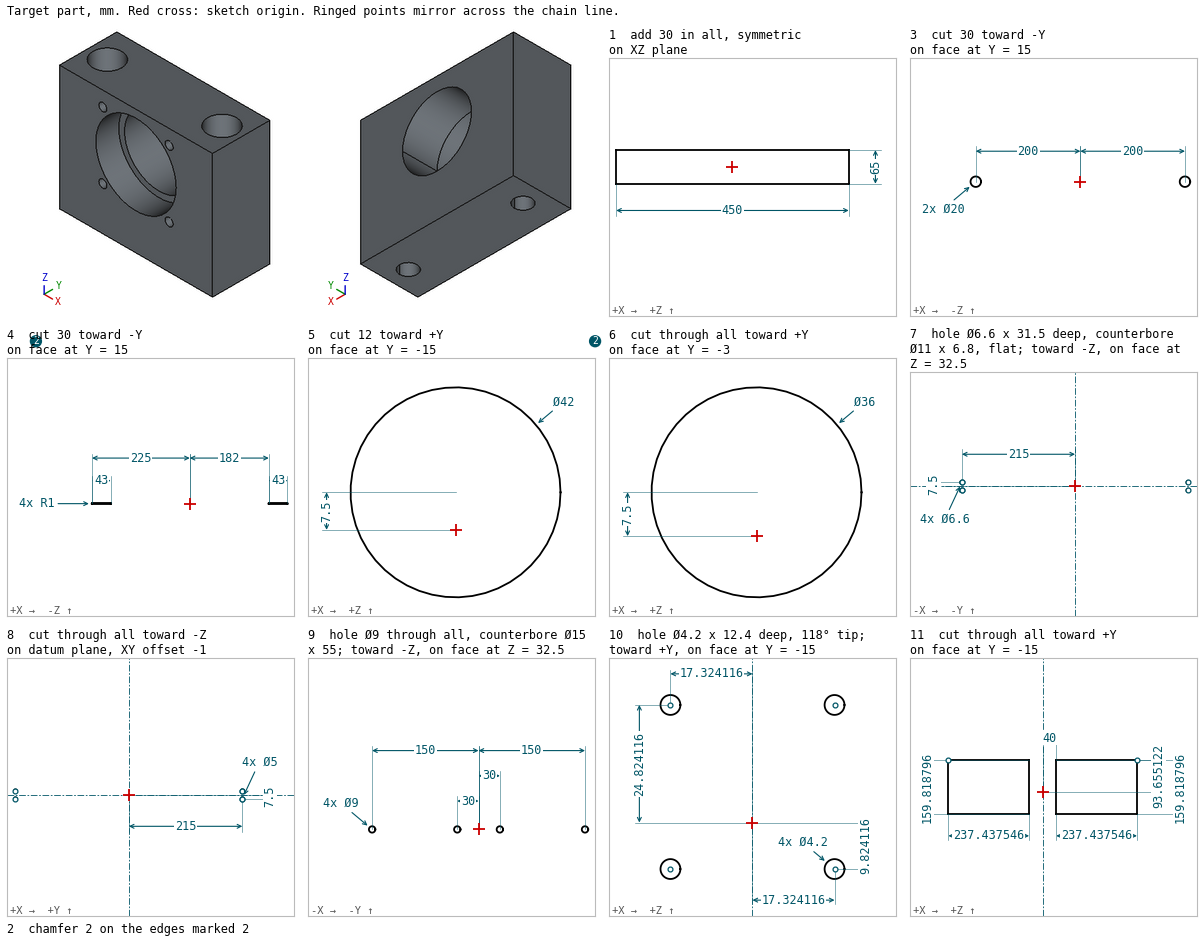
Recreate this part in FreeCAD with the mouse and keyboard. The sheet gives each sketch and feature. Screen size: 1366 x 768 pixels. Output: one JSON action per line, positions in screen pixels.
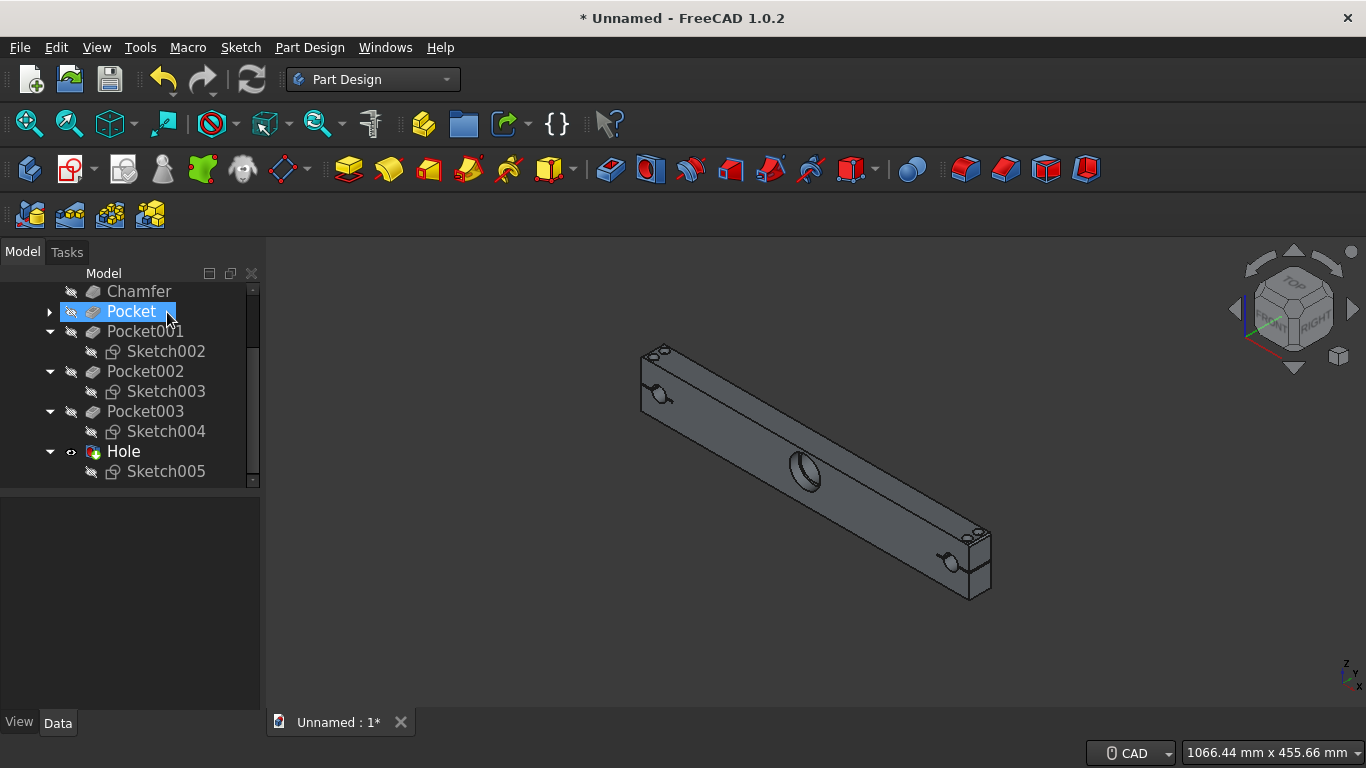
{"action": "key", "text": "1"}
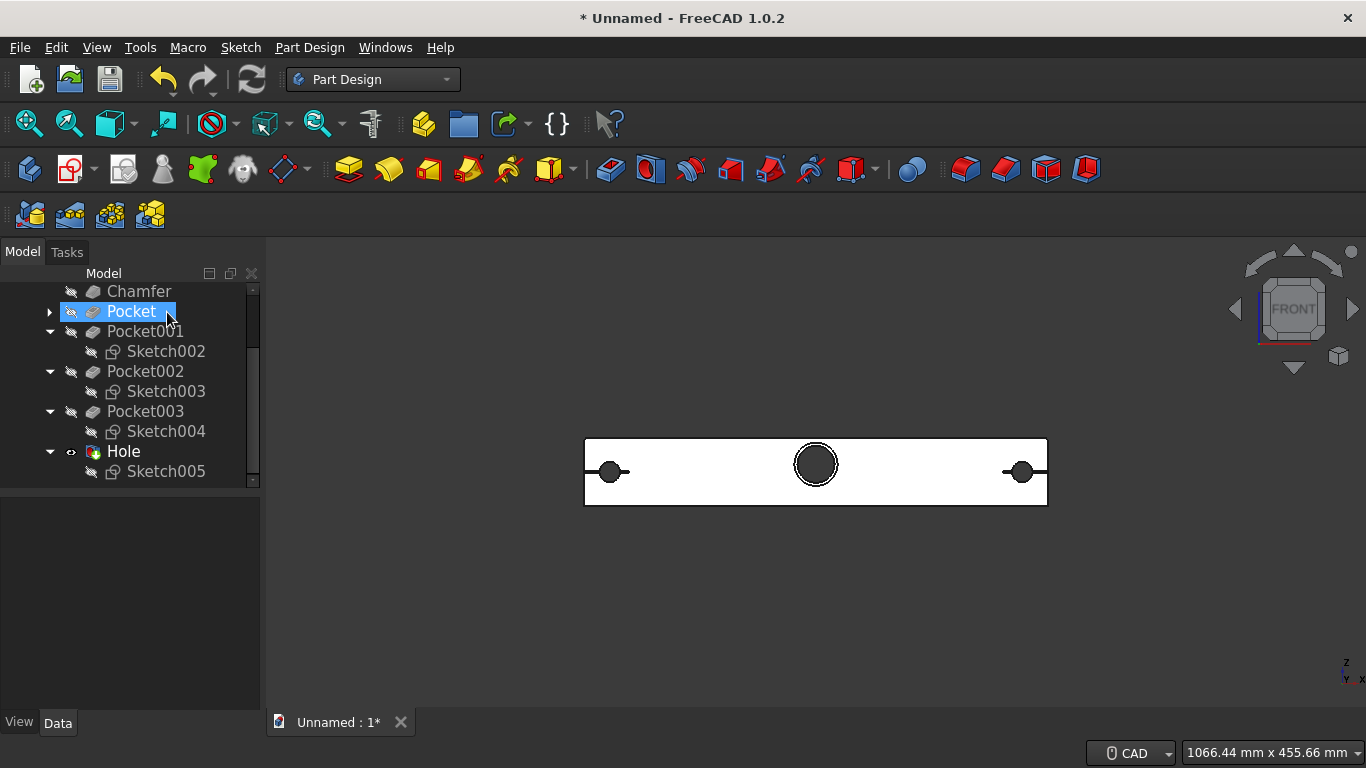
{"action": "key", "text": "v f"}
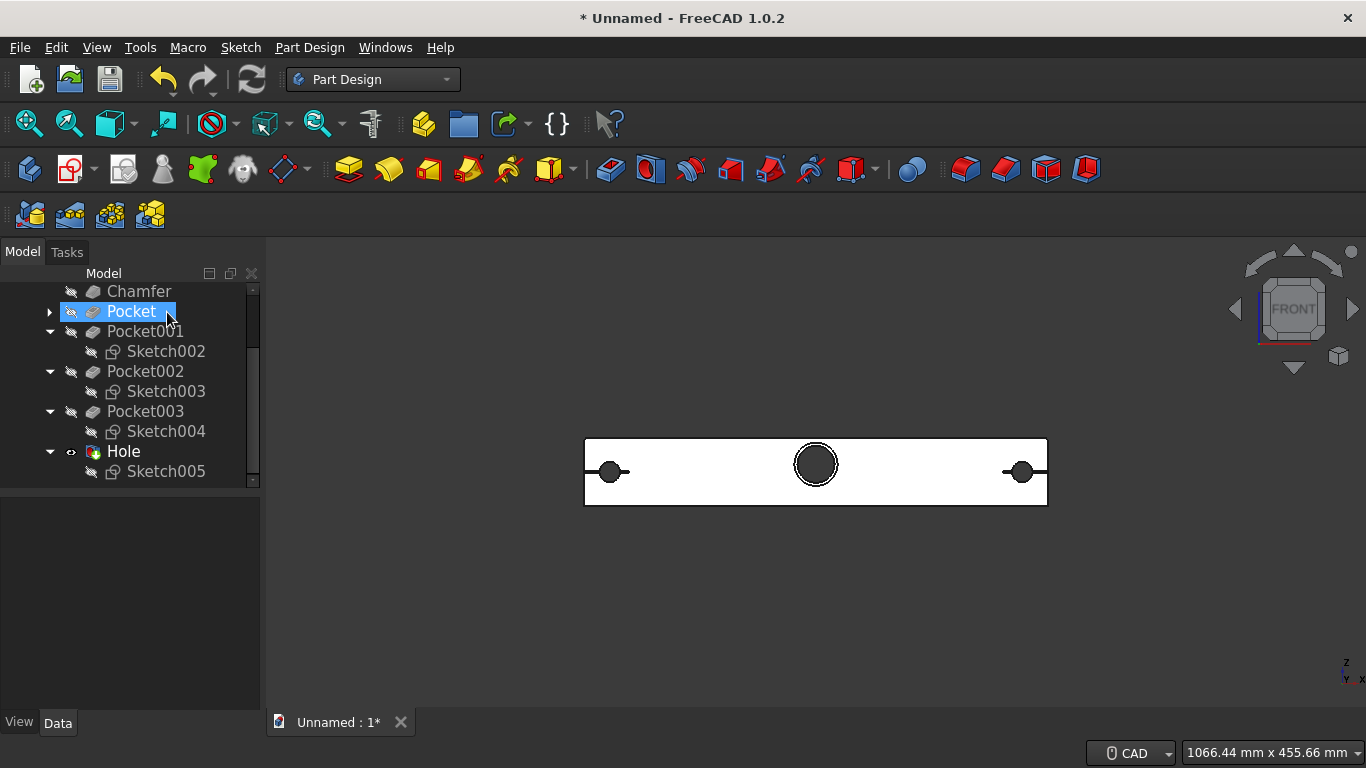
{"action": "scroll", "coordinate": [140, 387], "scroll_direction": "down", "scroll_amount": 3}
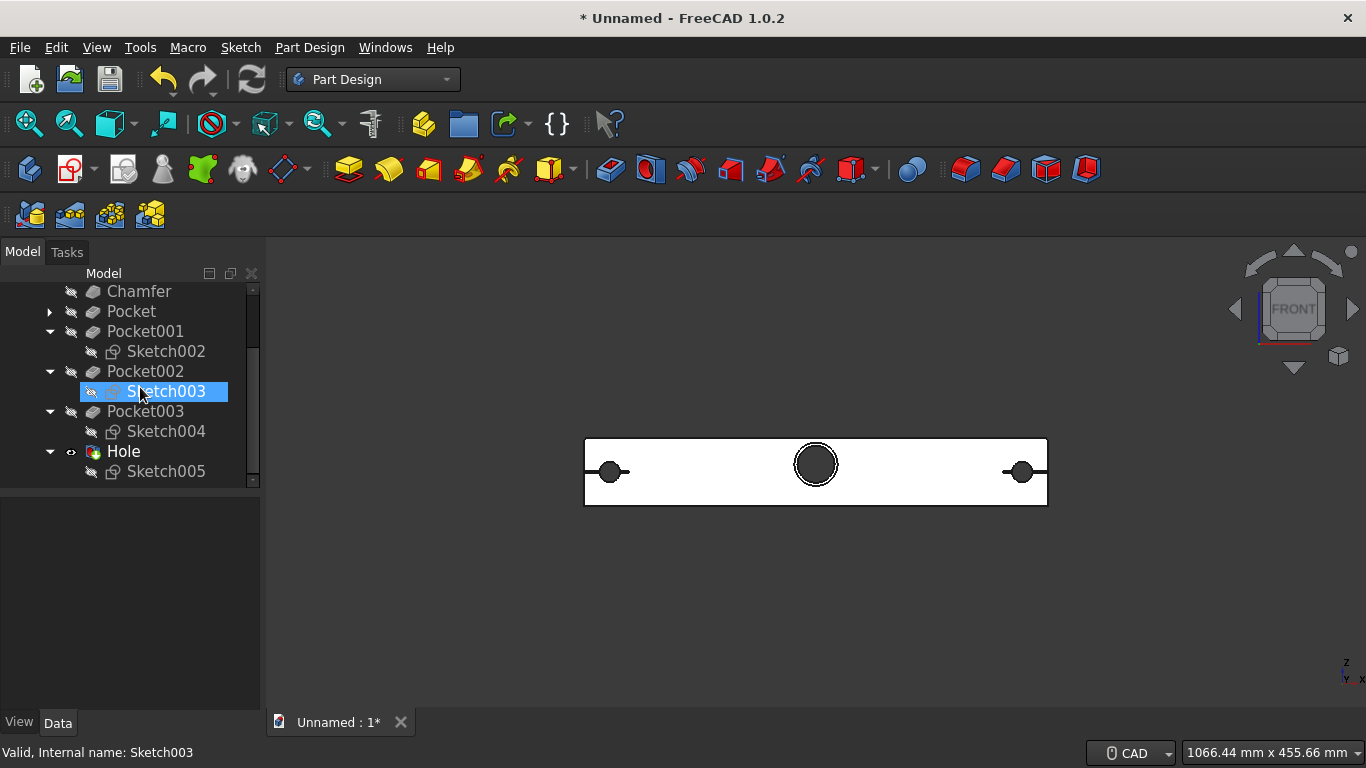
{"action": "scroll", "coordinate": [140, 387], "scroll_direction": "up", "scroll_amount": 15}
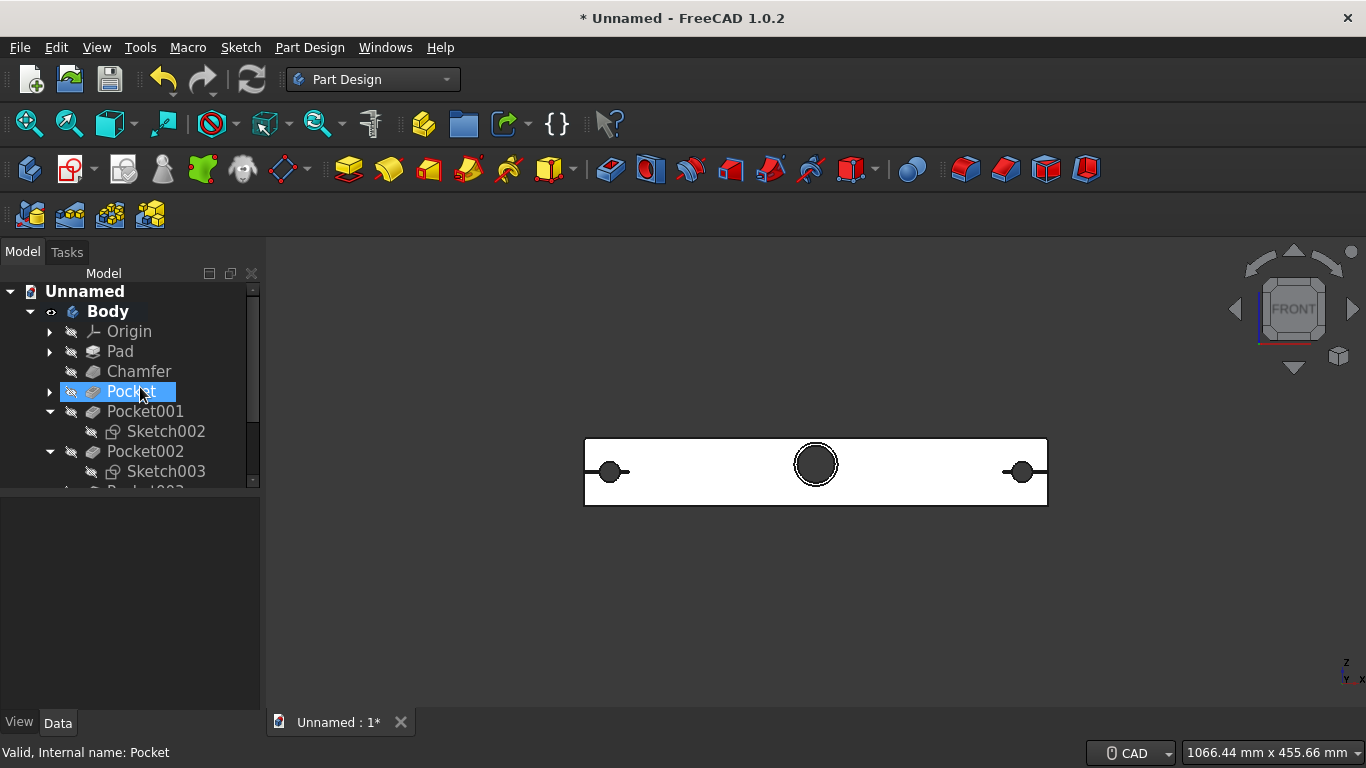
{"action": "left_click", "coordinate": [50, 332]}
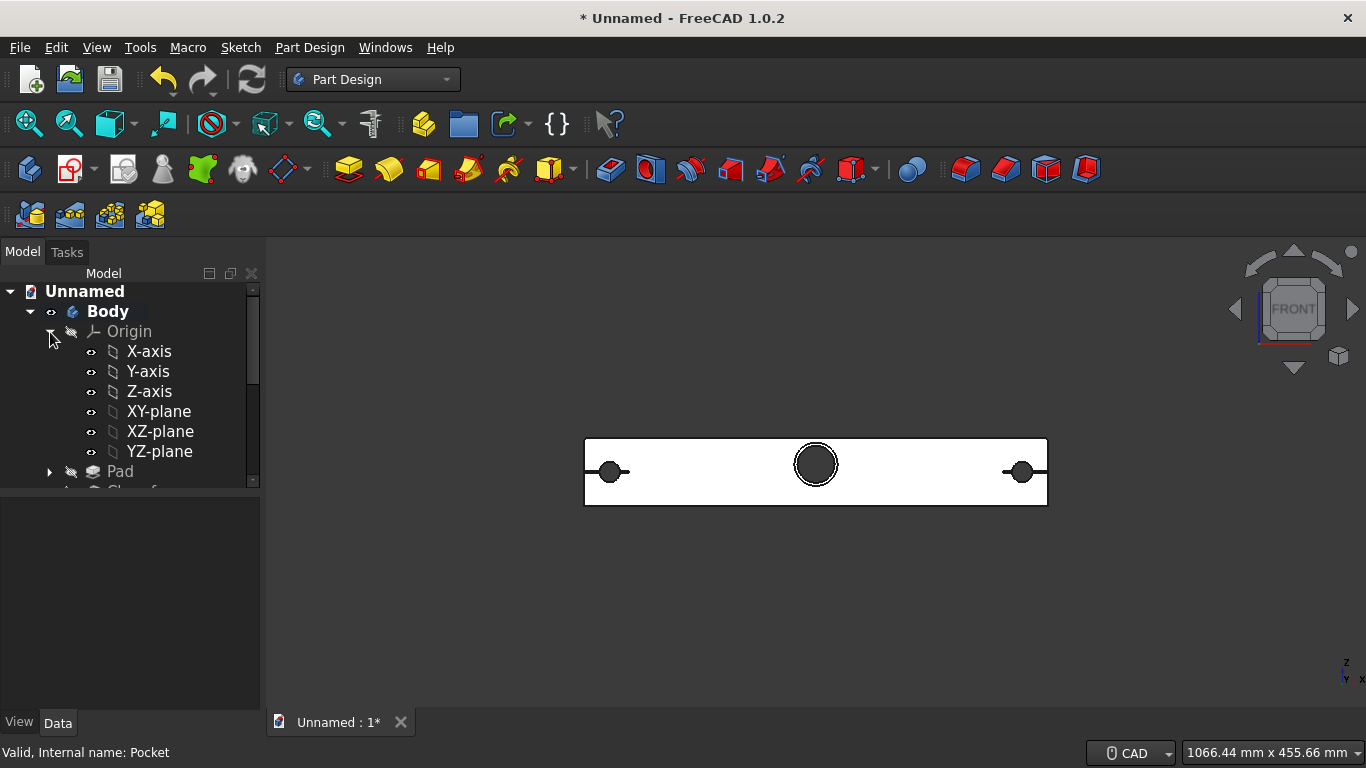
{"action": "left_click", "coordinate": [136, 412]}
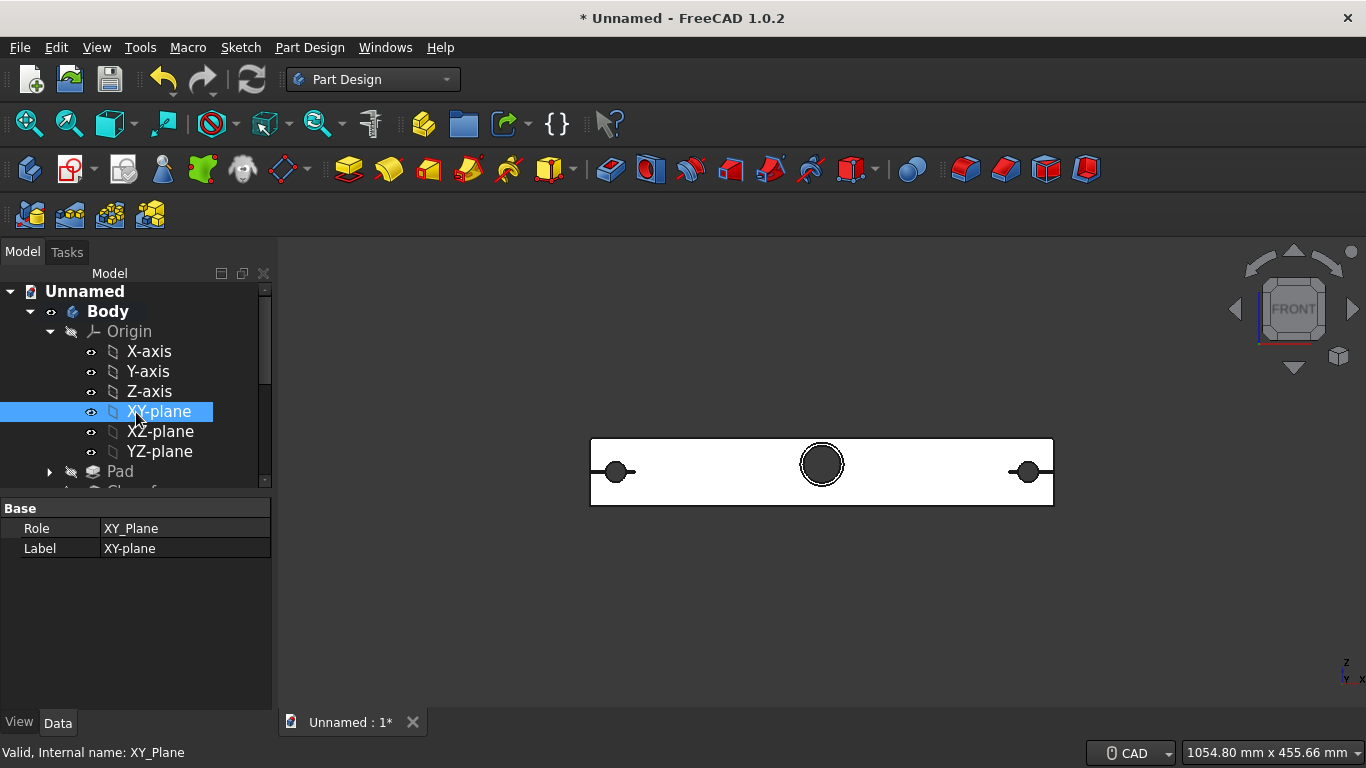
{"action": "left_click", "coordinate": [284, 170]}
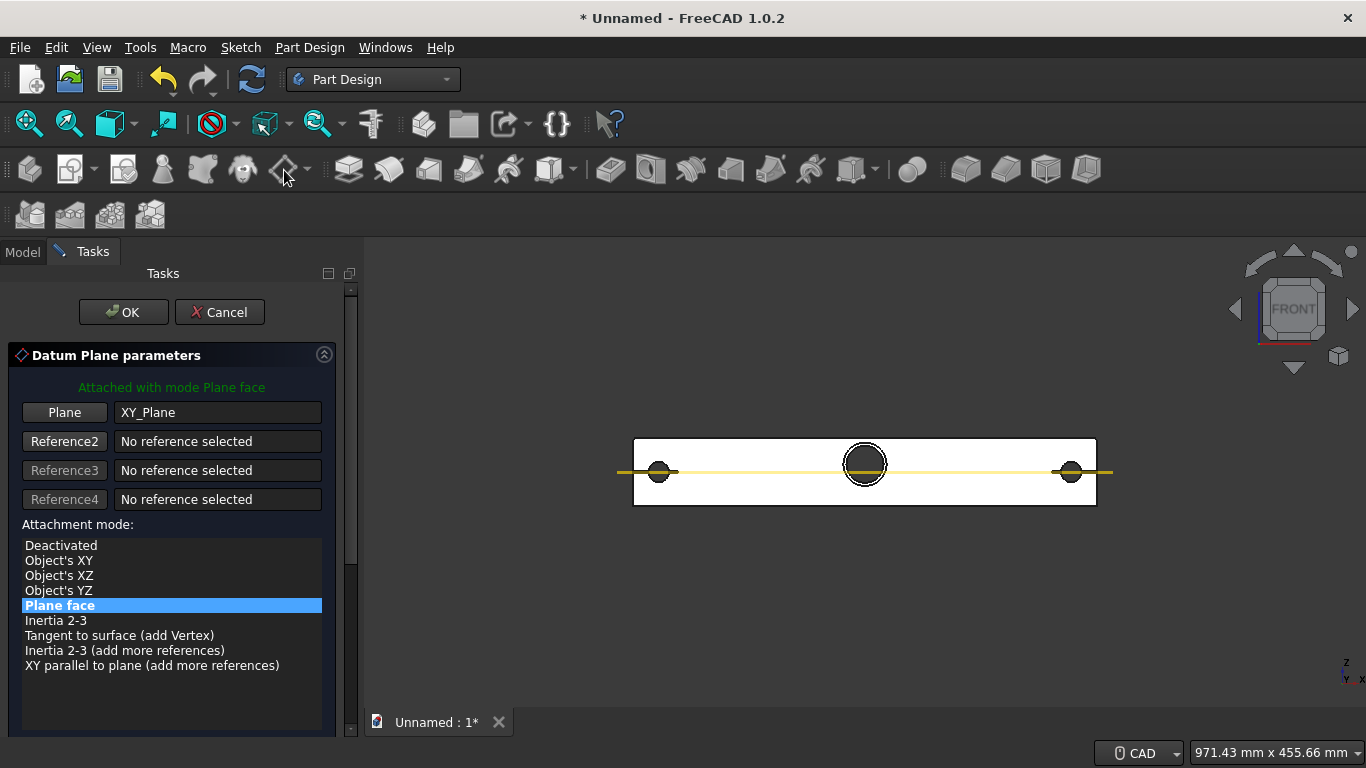
{"action": "scroll", "coordinate": [351, 510], "scroll_direction": "down", "scroll_amount": 3}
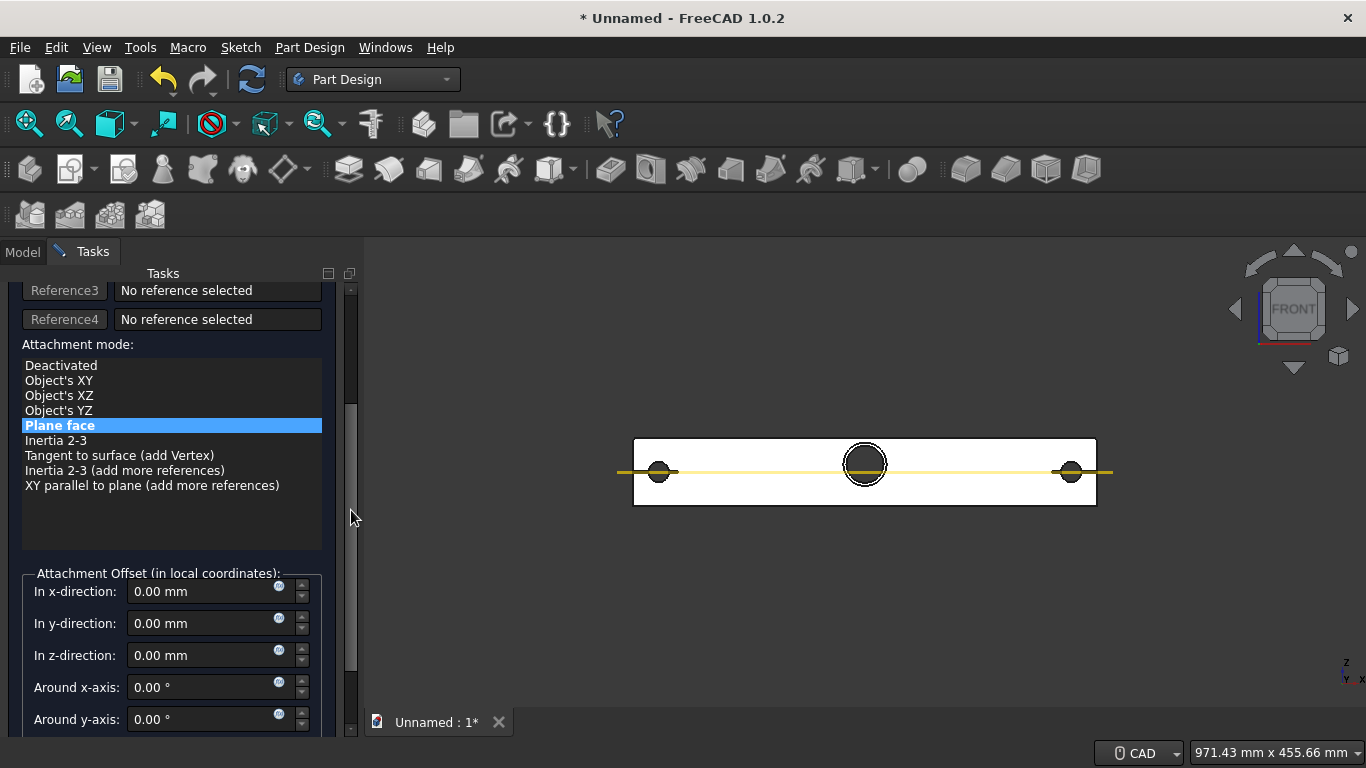
{"action": "triple_click", "coordinate": [210, 655]}